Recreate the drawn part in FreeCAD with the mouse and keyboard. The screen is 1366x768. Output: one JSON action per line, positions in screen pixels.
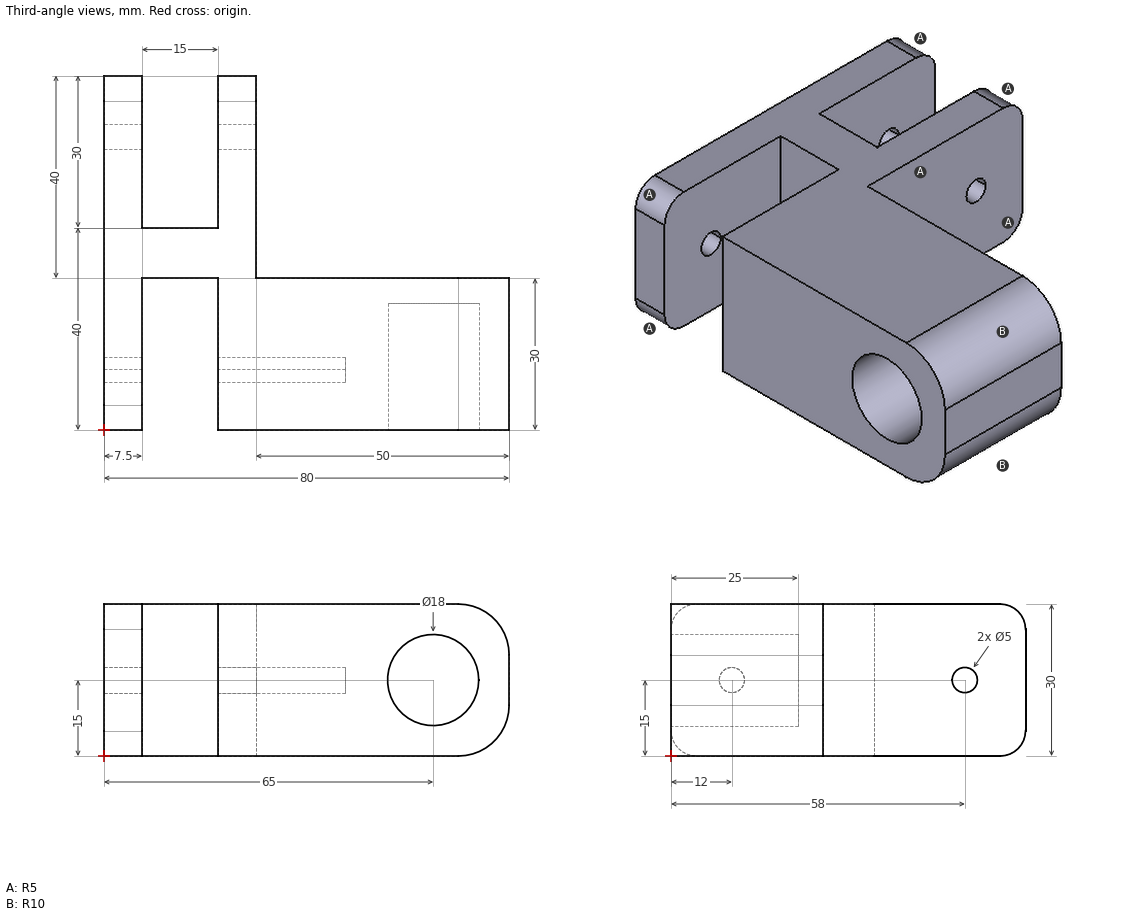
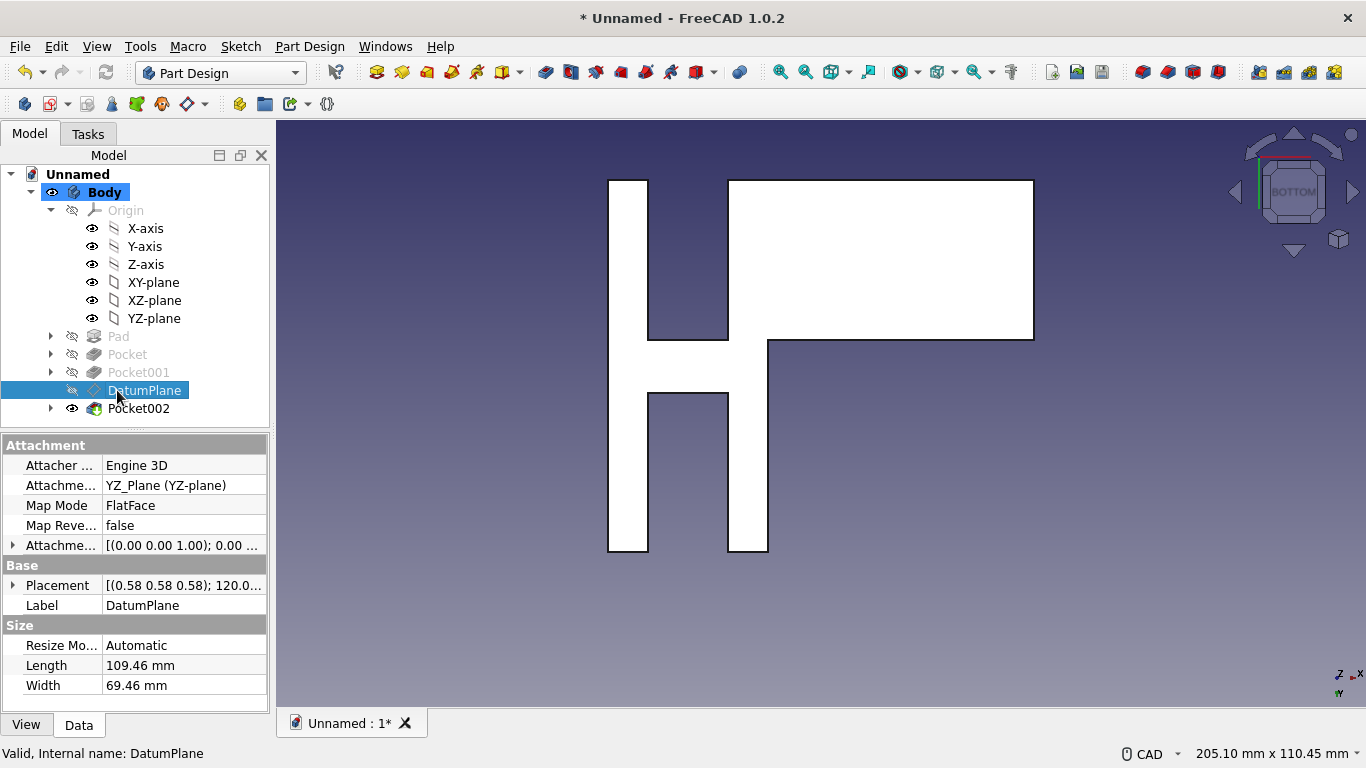
{"action": "left_click", "coordinate": [628, 551]}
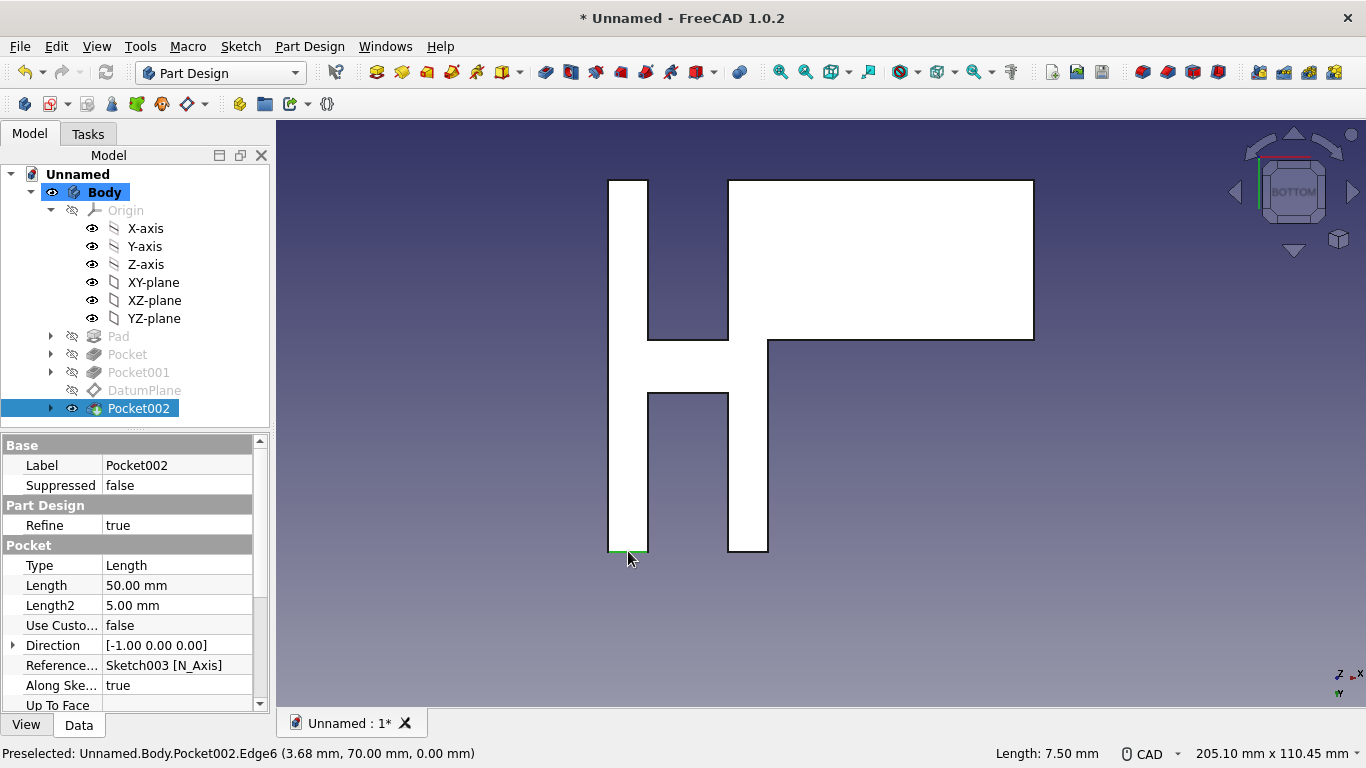
{"action": "left_click", "coordinate": [748, 551], "text": "ctrl"}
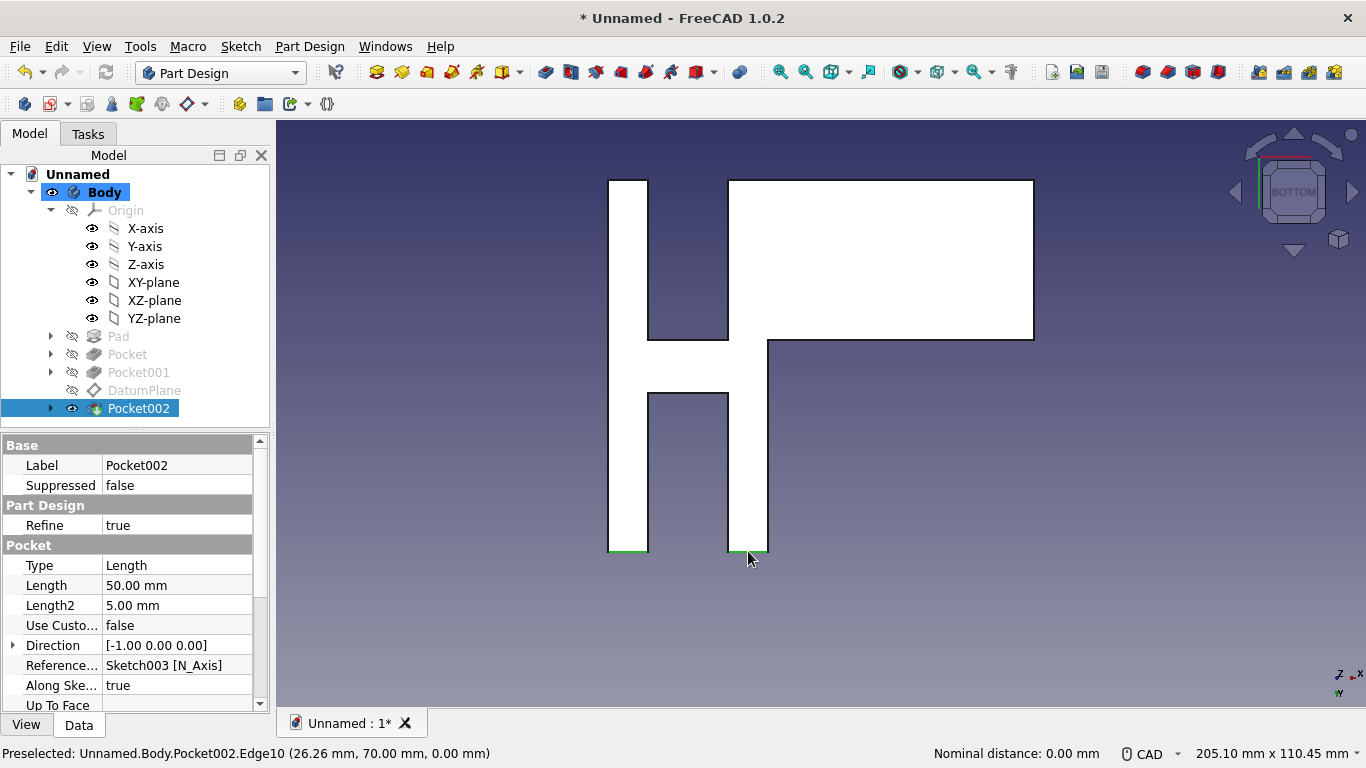
{"action": "key", "text": "0"}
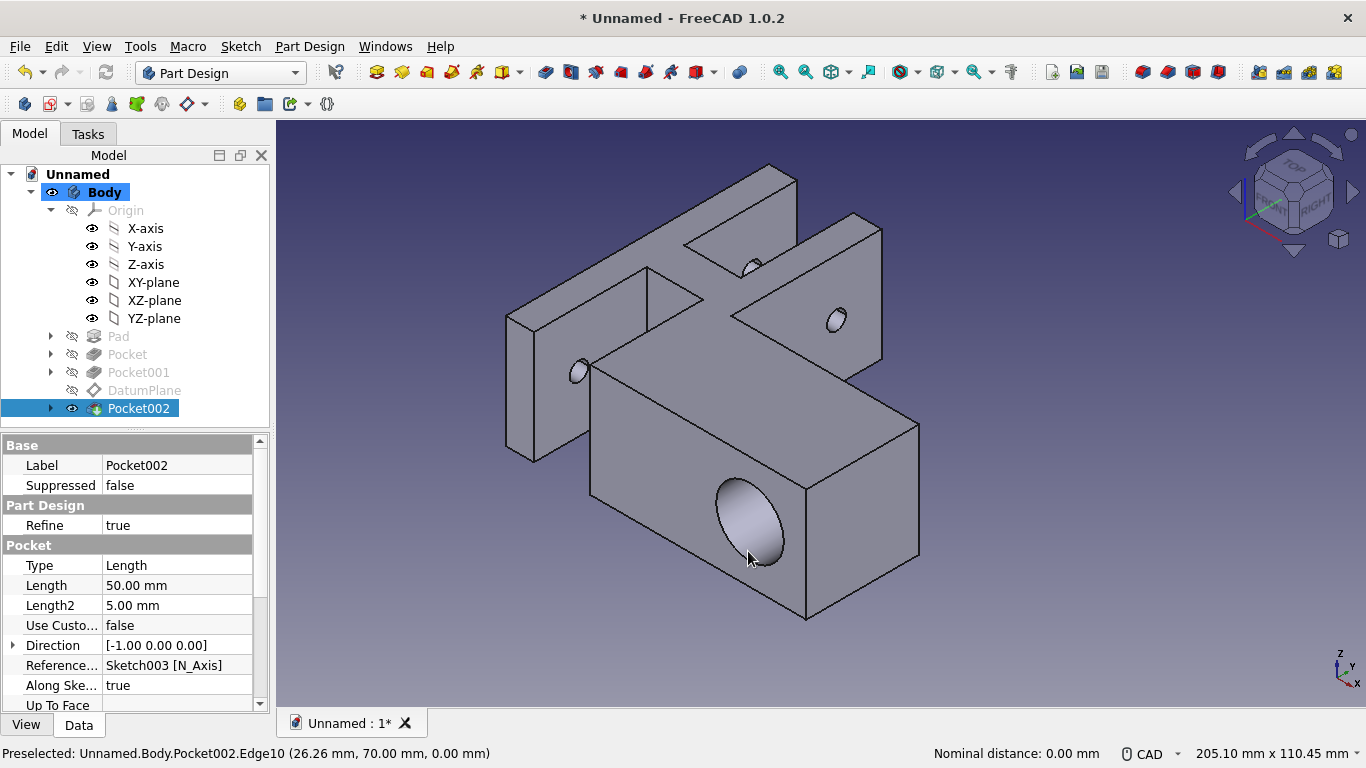
{"action": "left_click", "coordinate": [520, 323], "text": "ctrl"}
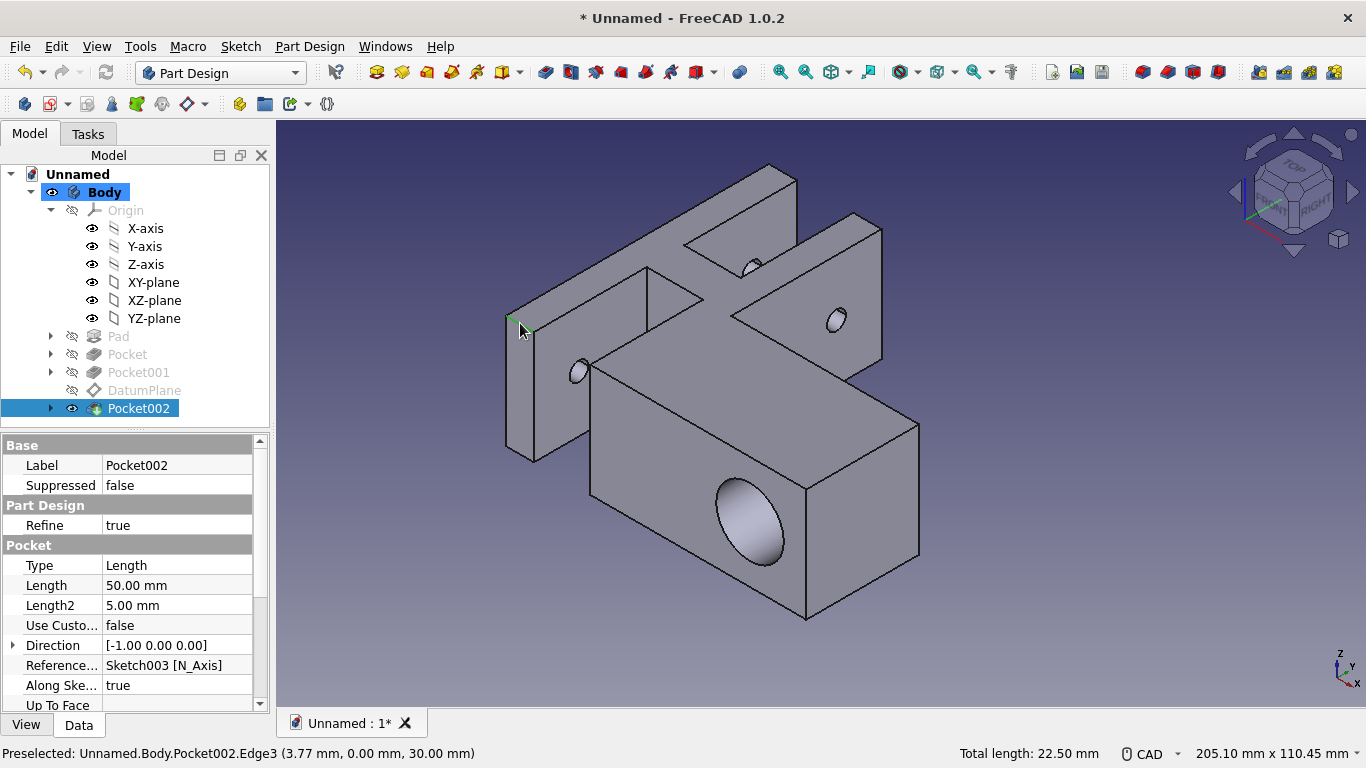
{"action": "key", "text": "2"}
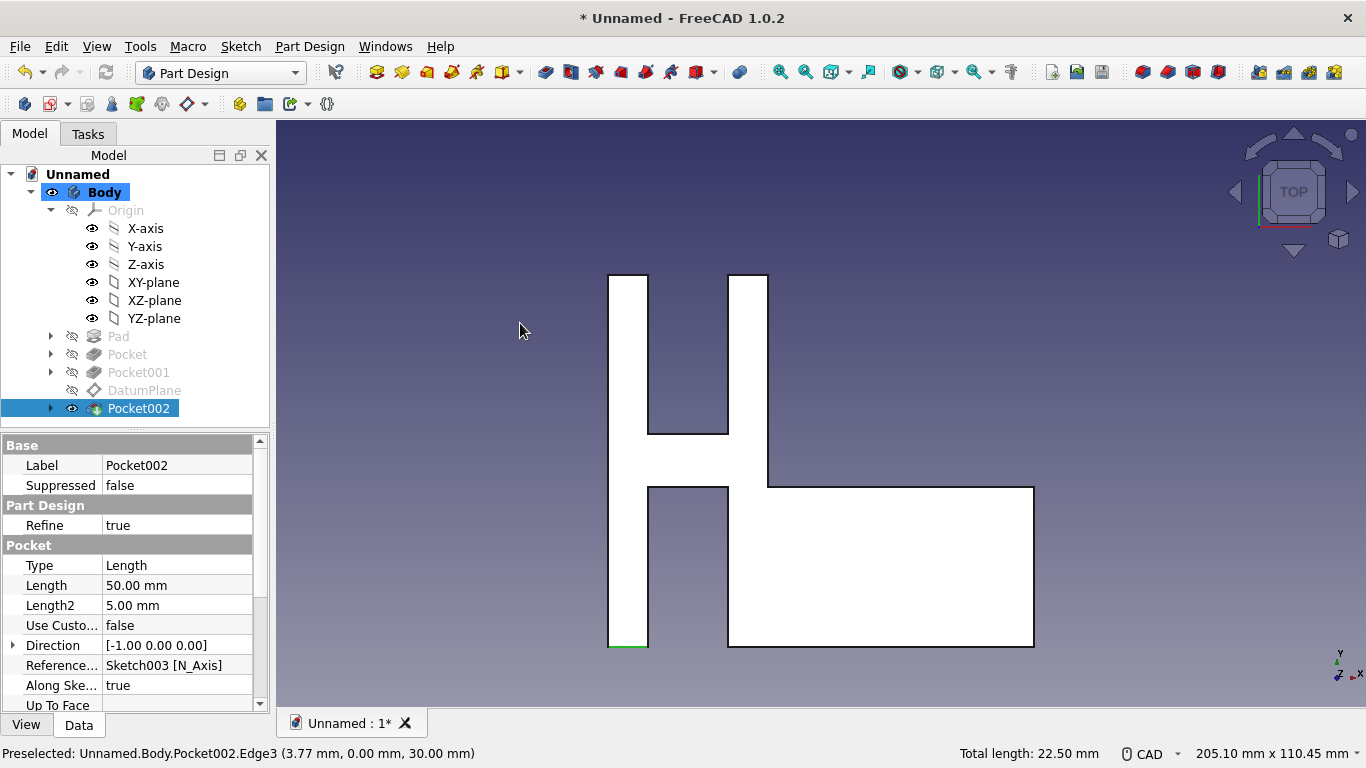
{"action": "left_click", "coordinate": [748, 274], "text": "ctrl"}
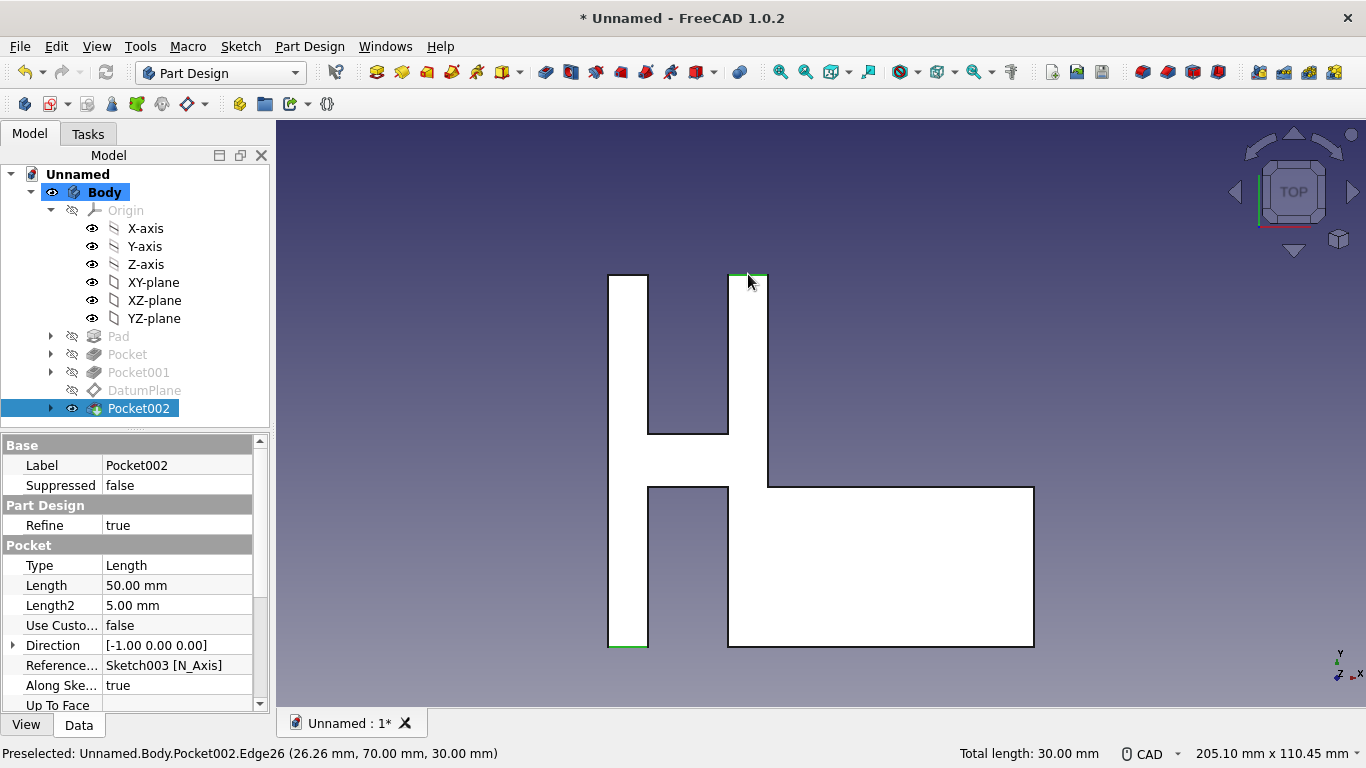
{"action": "left_click", "coordinate": [628, 274], "text": "ctrl"}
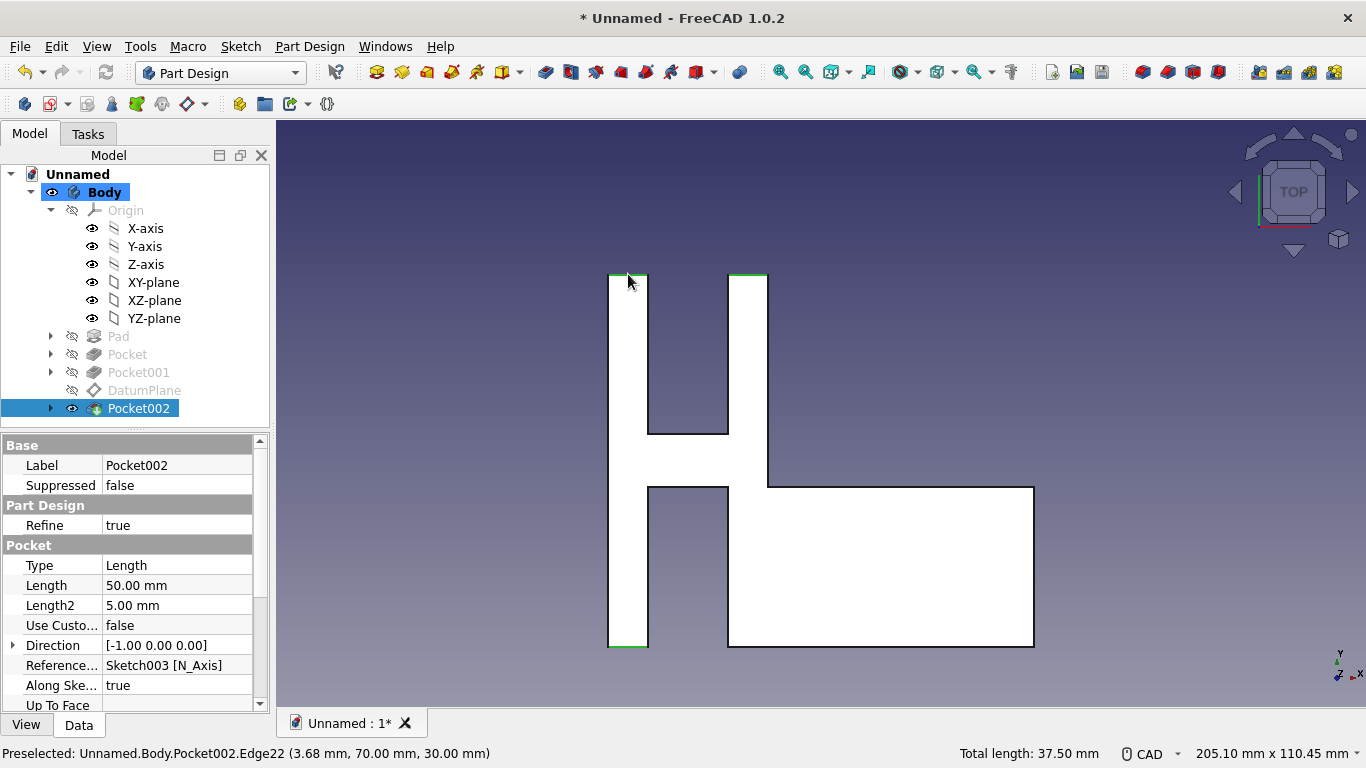
{"action": "key", "text": "1"}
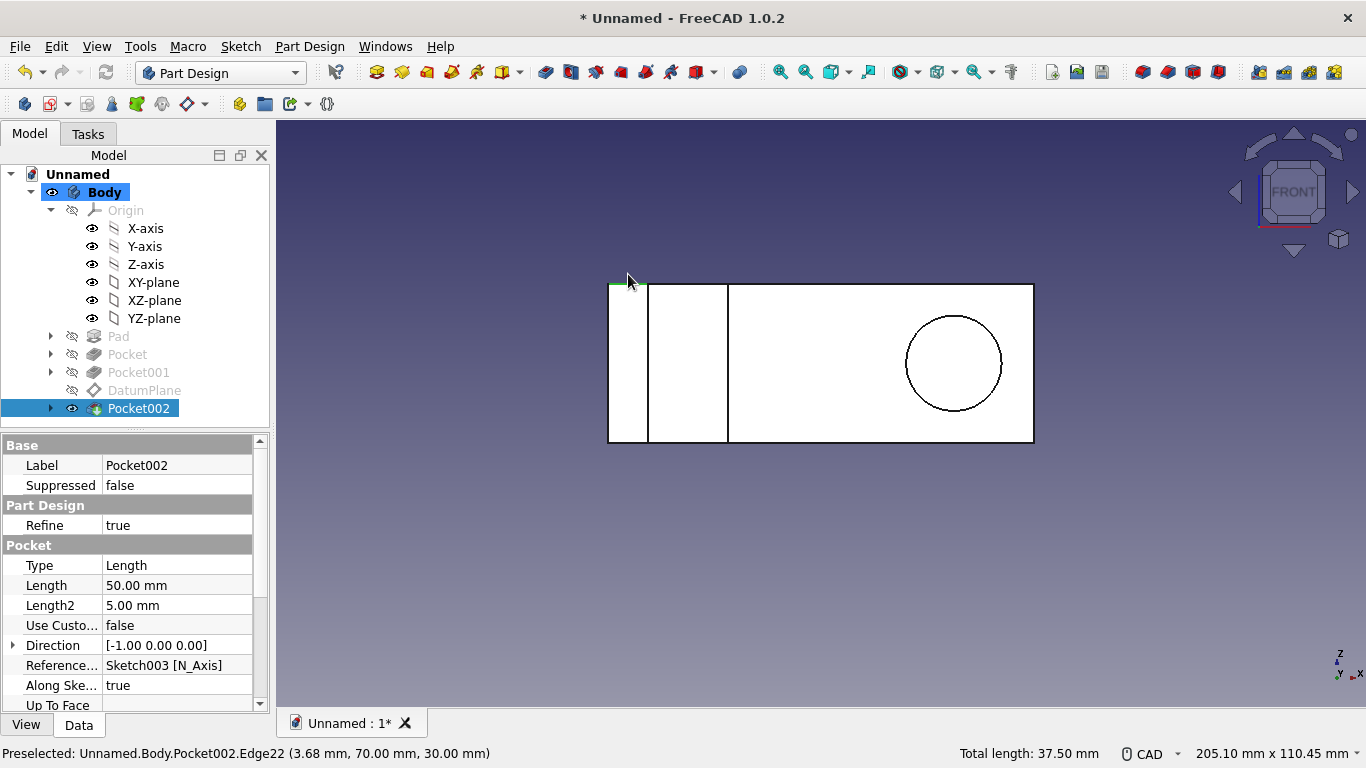
{"action": "key", "text": "v f"}